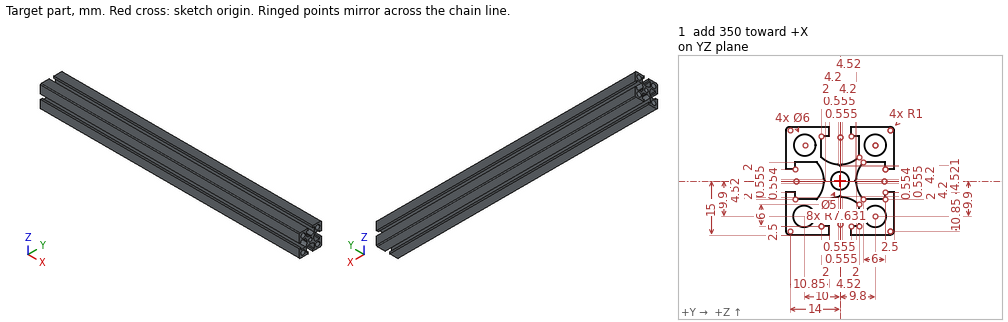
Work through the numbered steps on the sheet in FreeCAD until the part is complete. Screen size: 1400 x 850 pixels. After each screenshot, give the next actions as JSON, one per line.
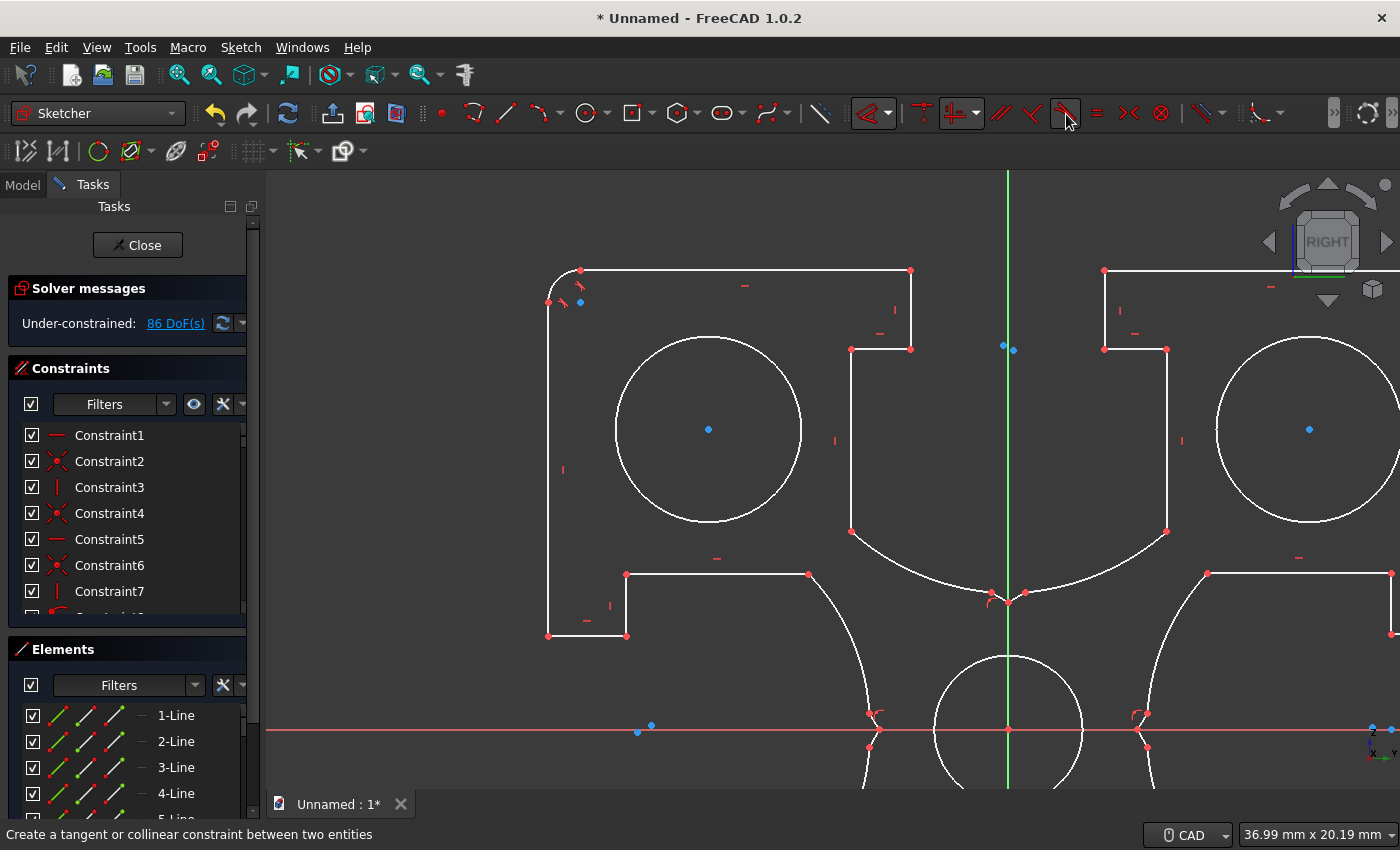
{"action": "scroll", "coordinate": [565, 275], "scroll_direction": "down", "scroll_amount": 4}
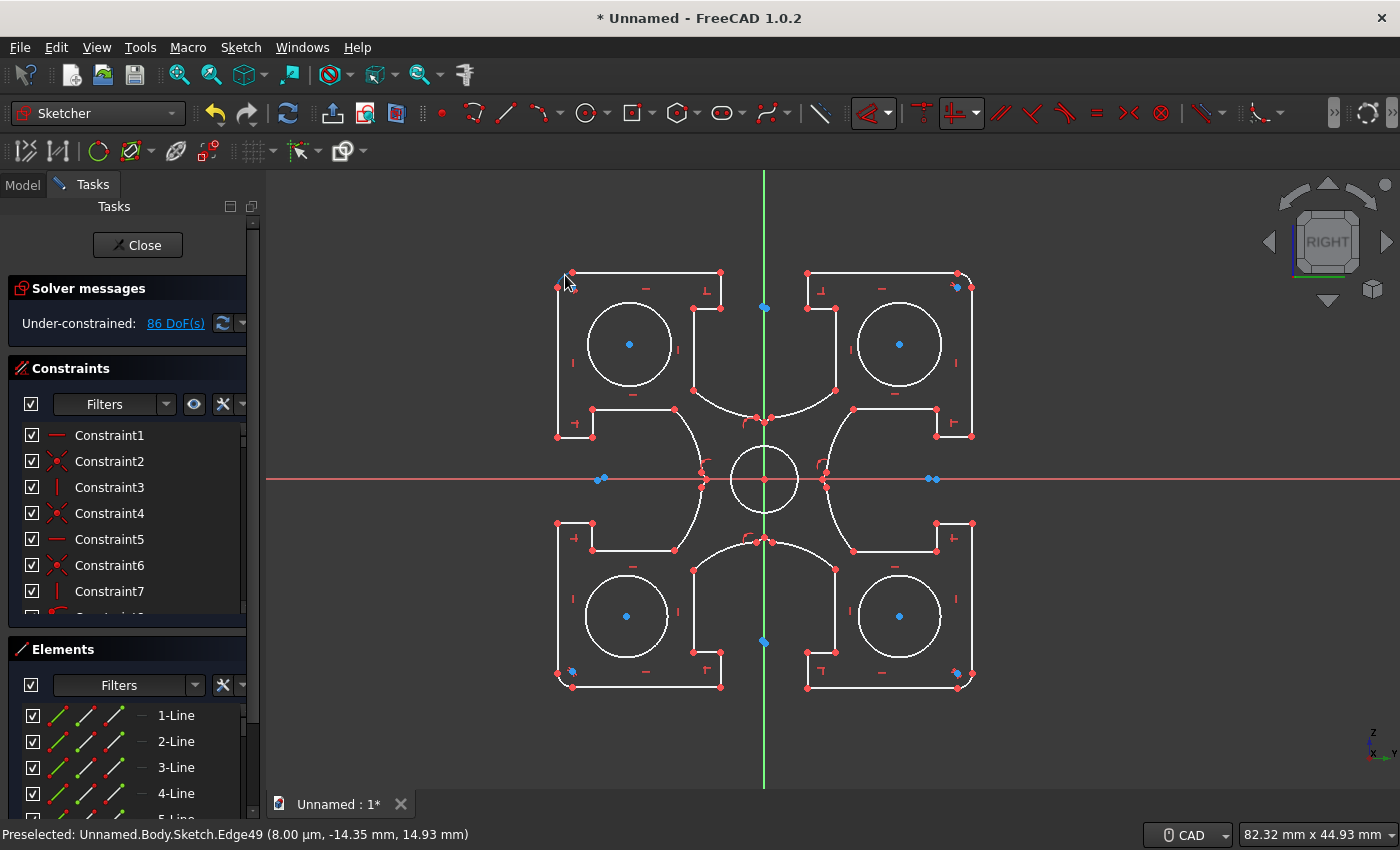
{"action": "left_click", "coordinate": [558, 568]}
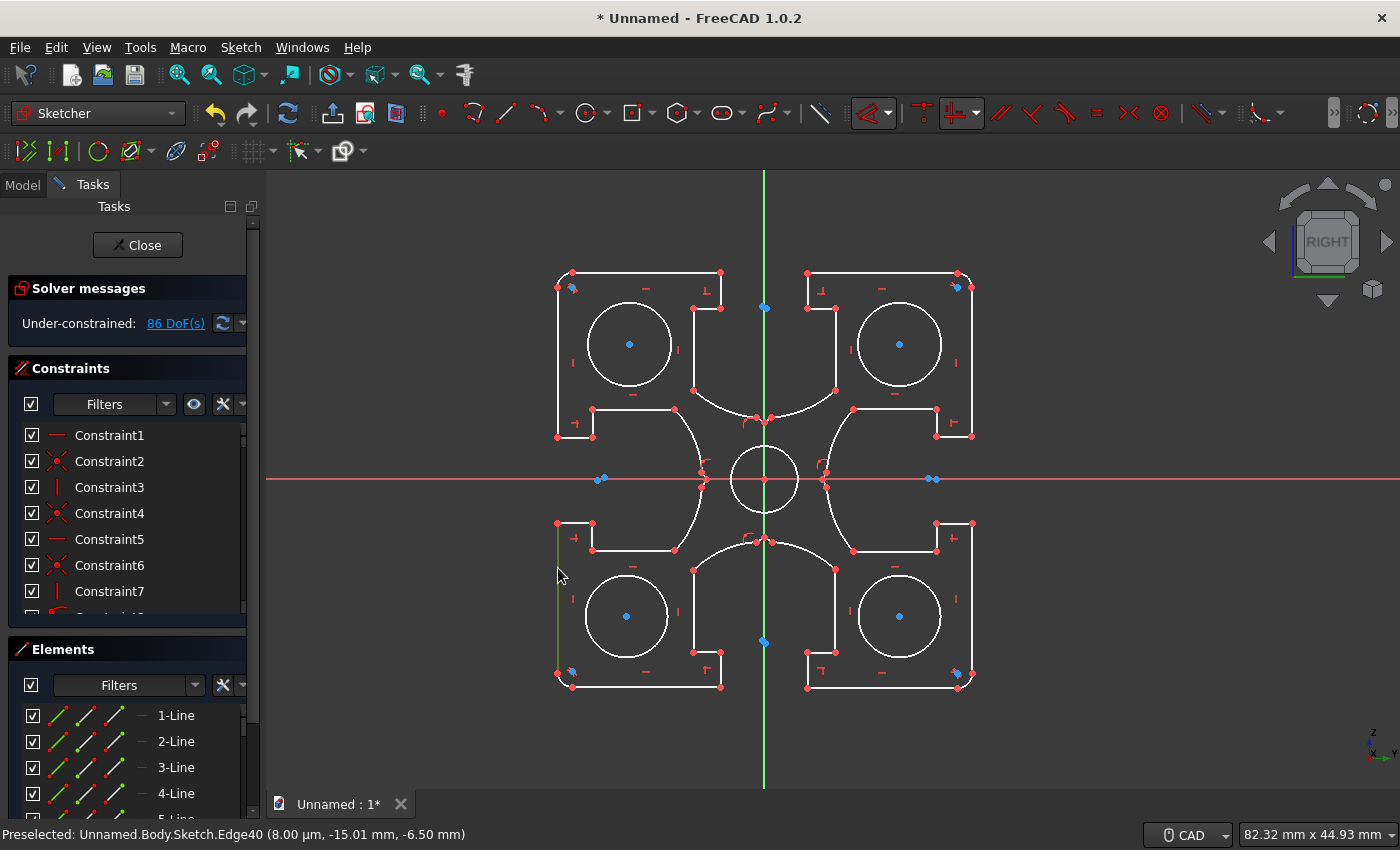
{"action": "scroll", "coordinate": [563, 683], "scroll_direction": "up", "scroll_amount": 2}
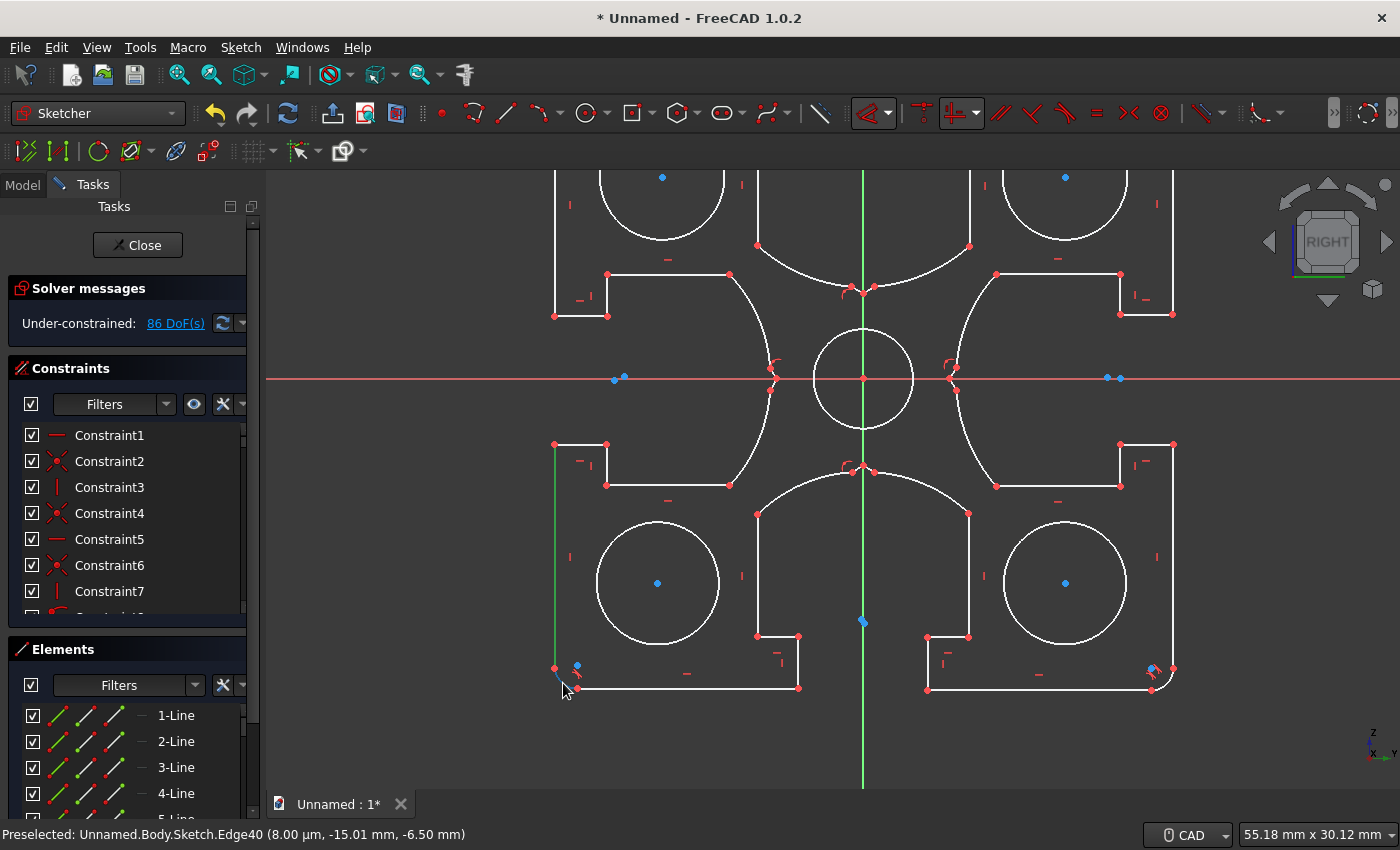
{"action": "left_click", "coordinate": [562, 683]}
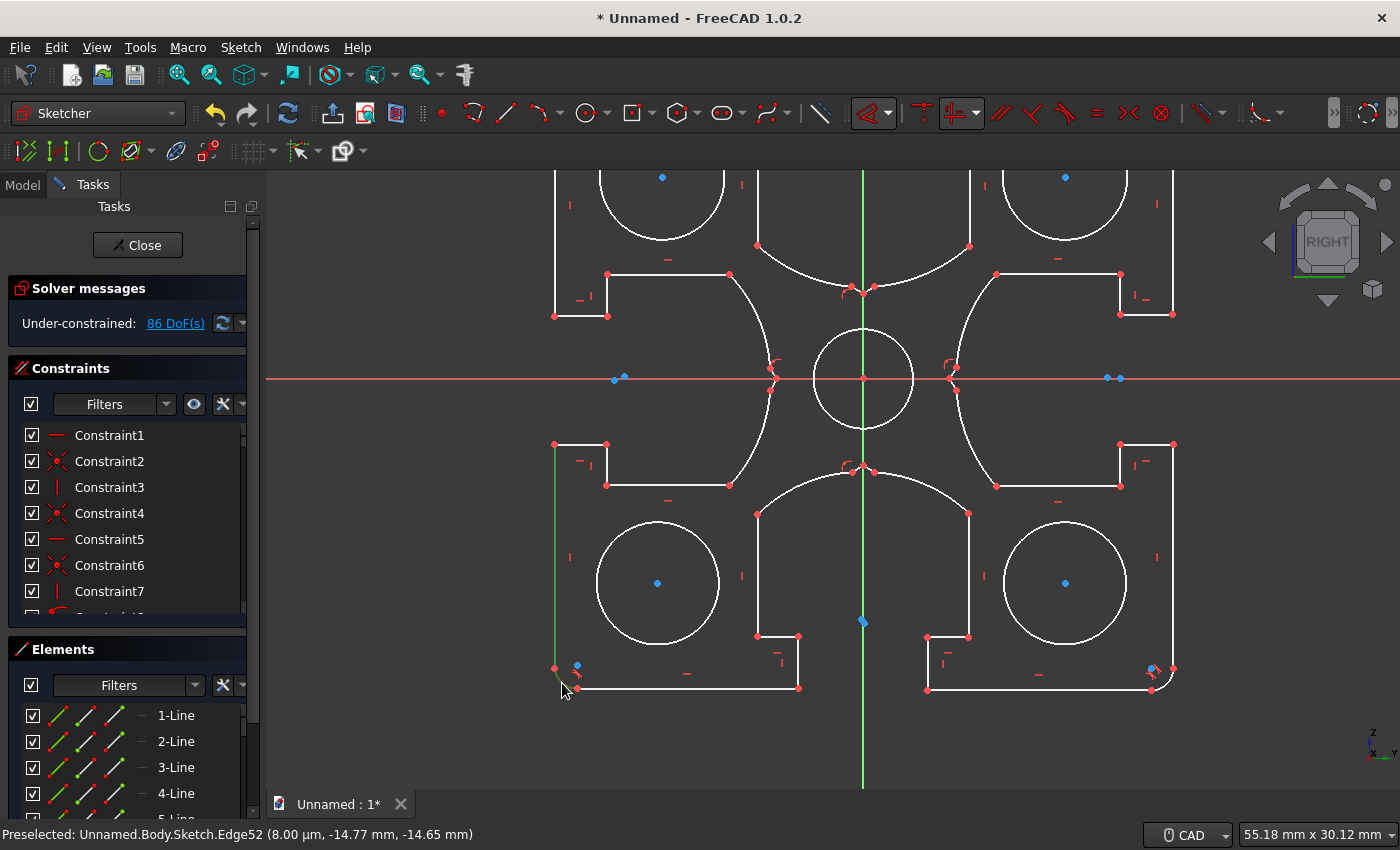
{"action": "left_click", "coordinate": [1066, 114]}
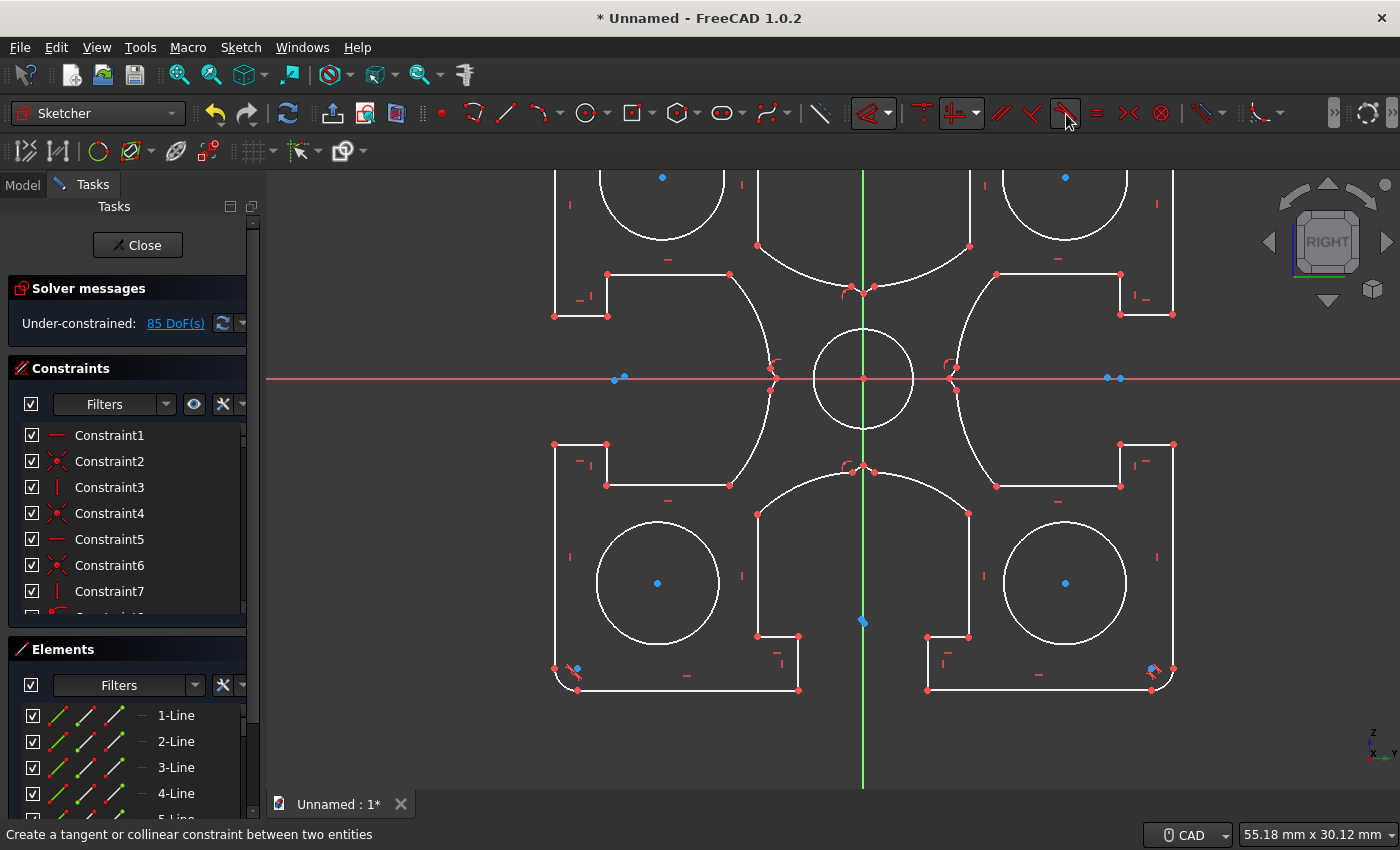
{"action": "left_click", "coordinate": [821, 478]}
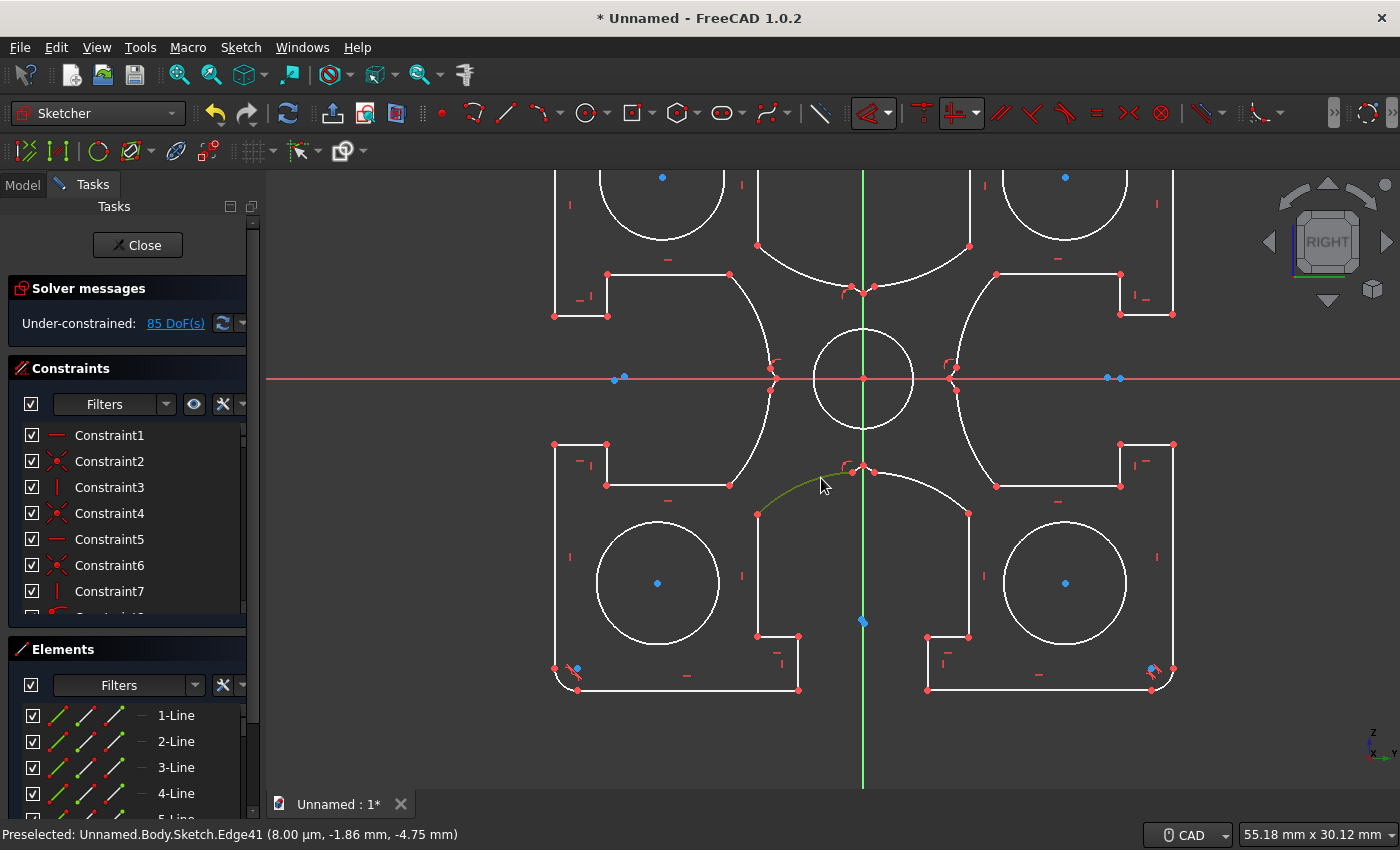
{"action": "left_click", "coordinate": [944, 494]}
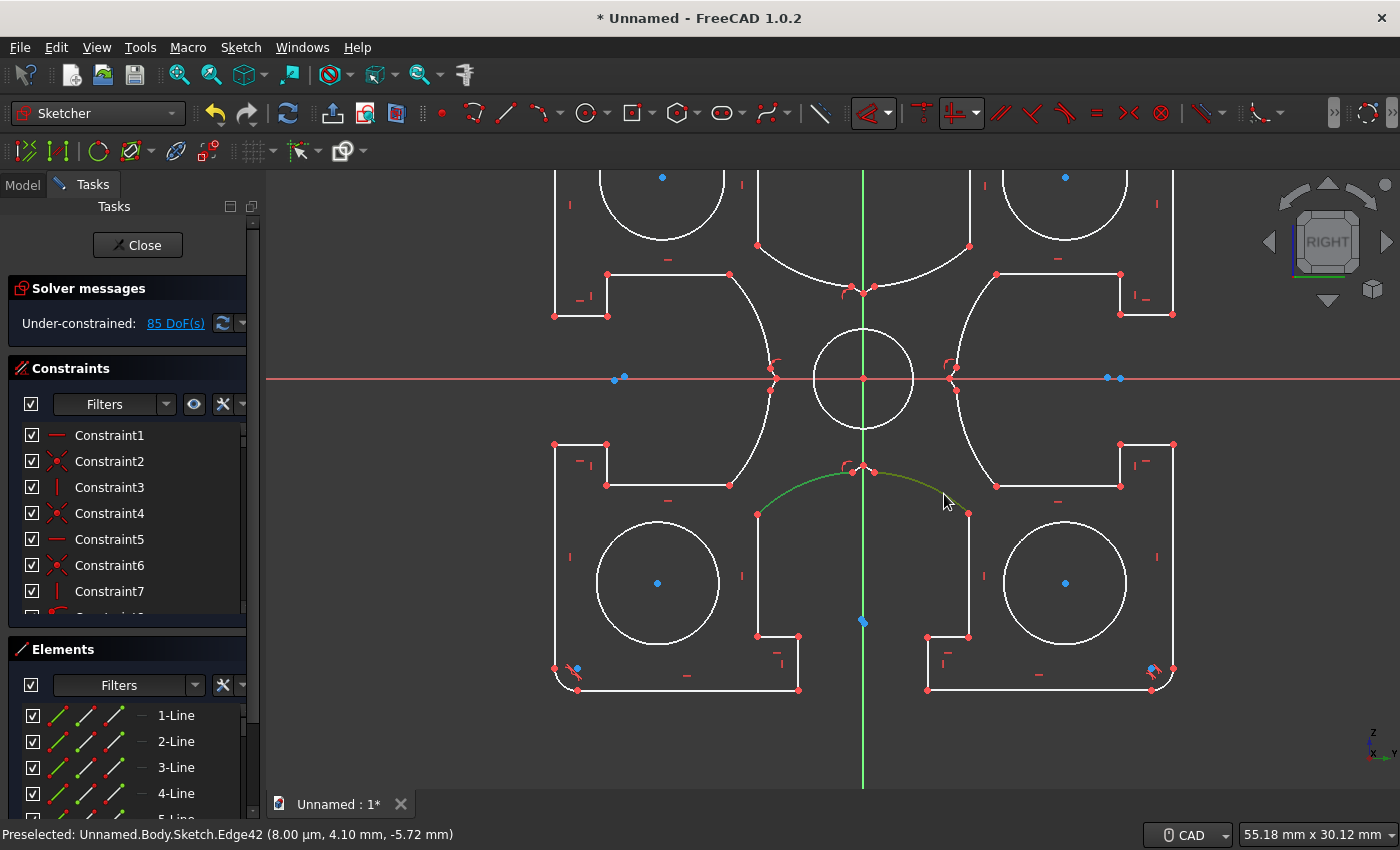
{"action": "left_click", "coordinate": [962, 422]}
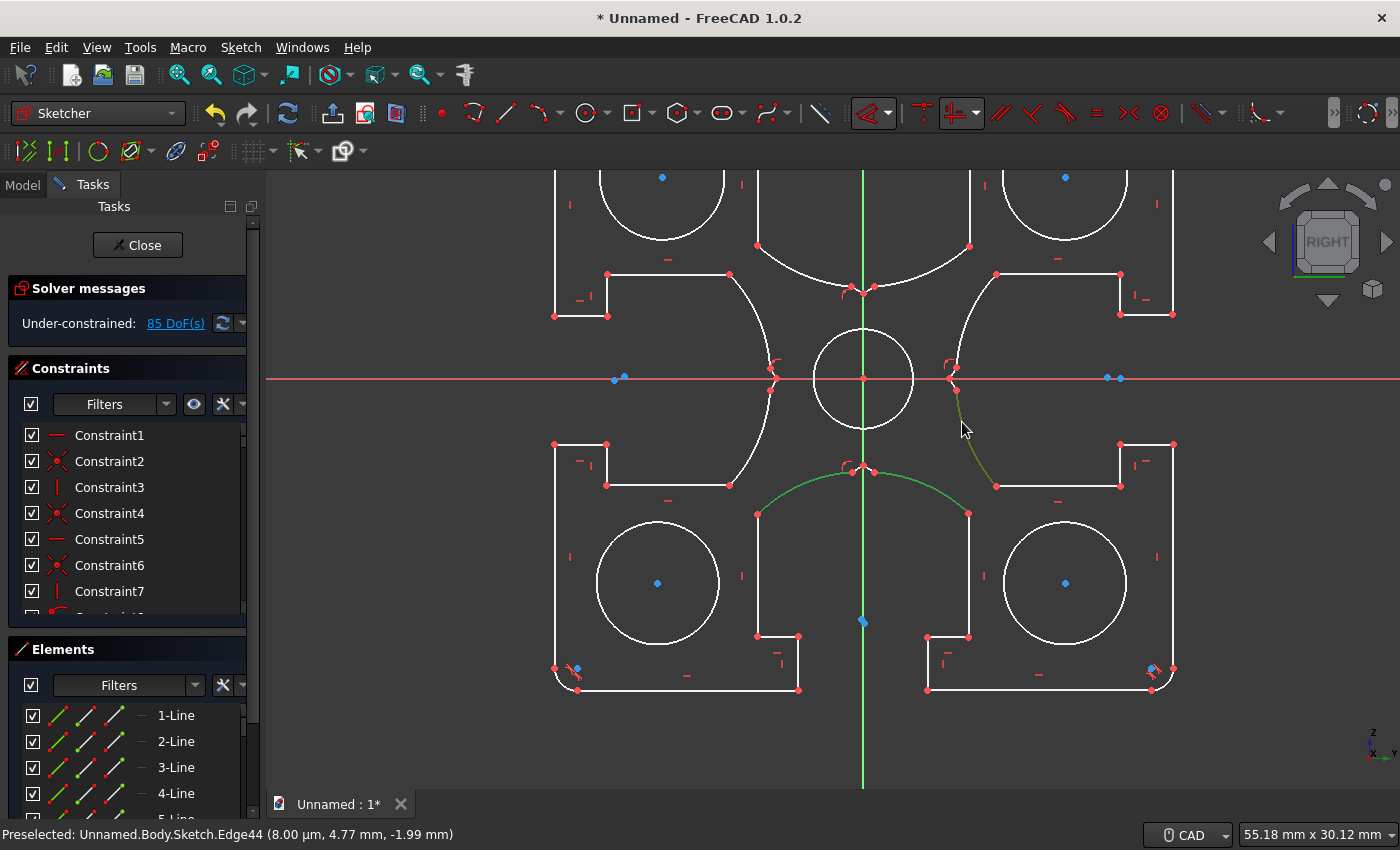
{"action": "left_click", "coordinate": [978, 299]}